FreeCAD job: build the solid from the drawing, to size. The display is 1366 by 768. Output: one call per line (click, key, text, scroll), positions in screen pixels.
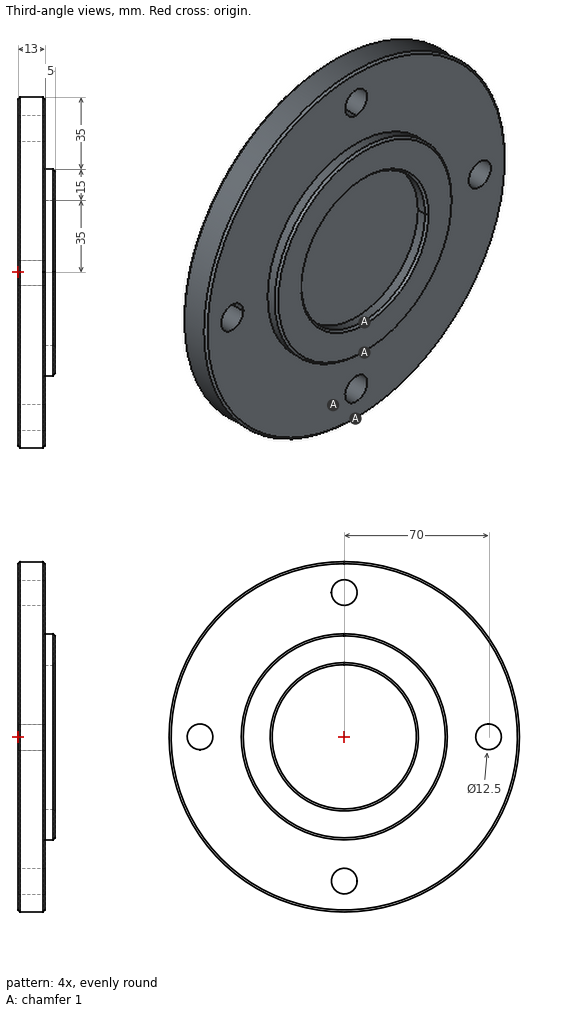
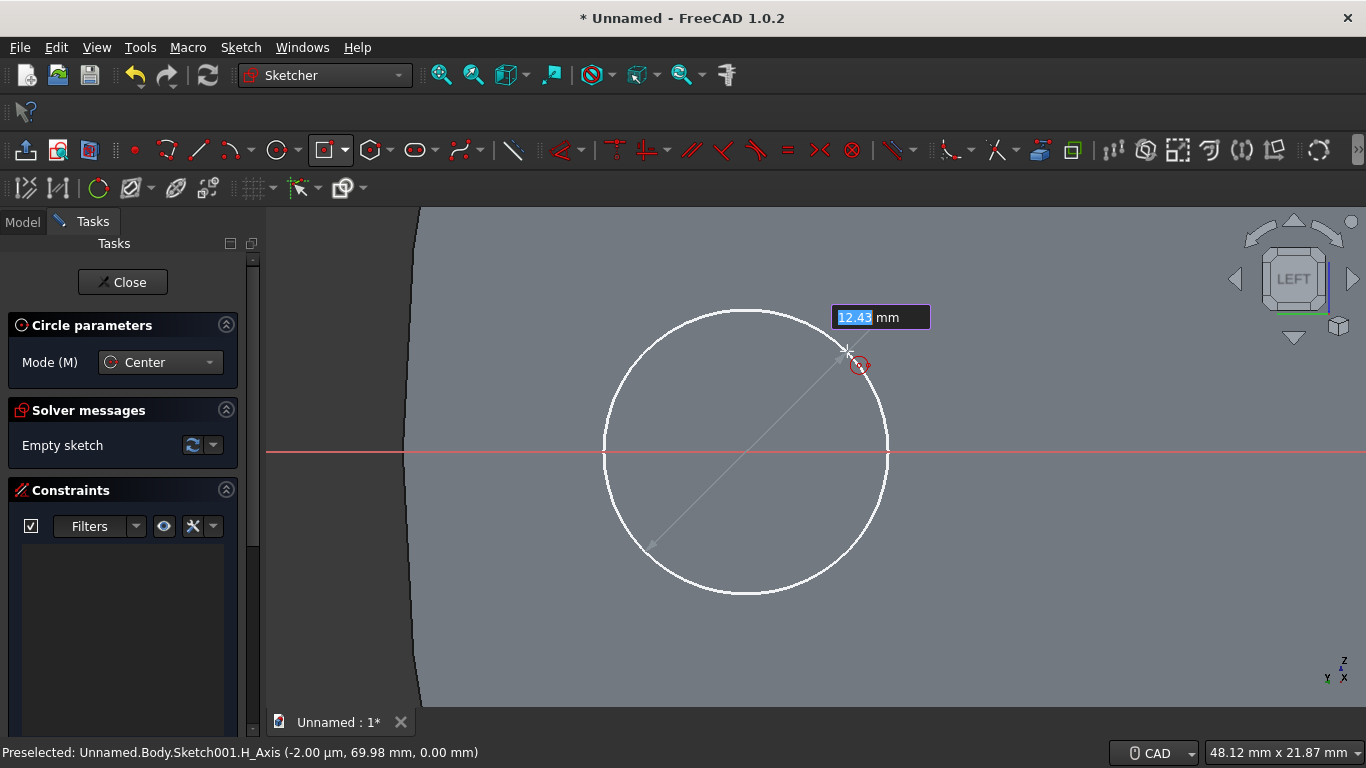
text(12.5)
key(Return)
key(Escape)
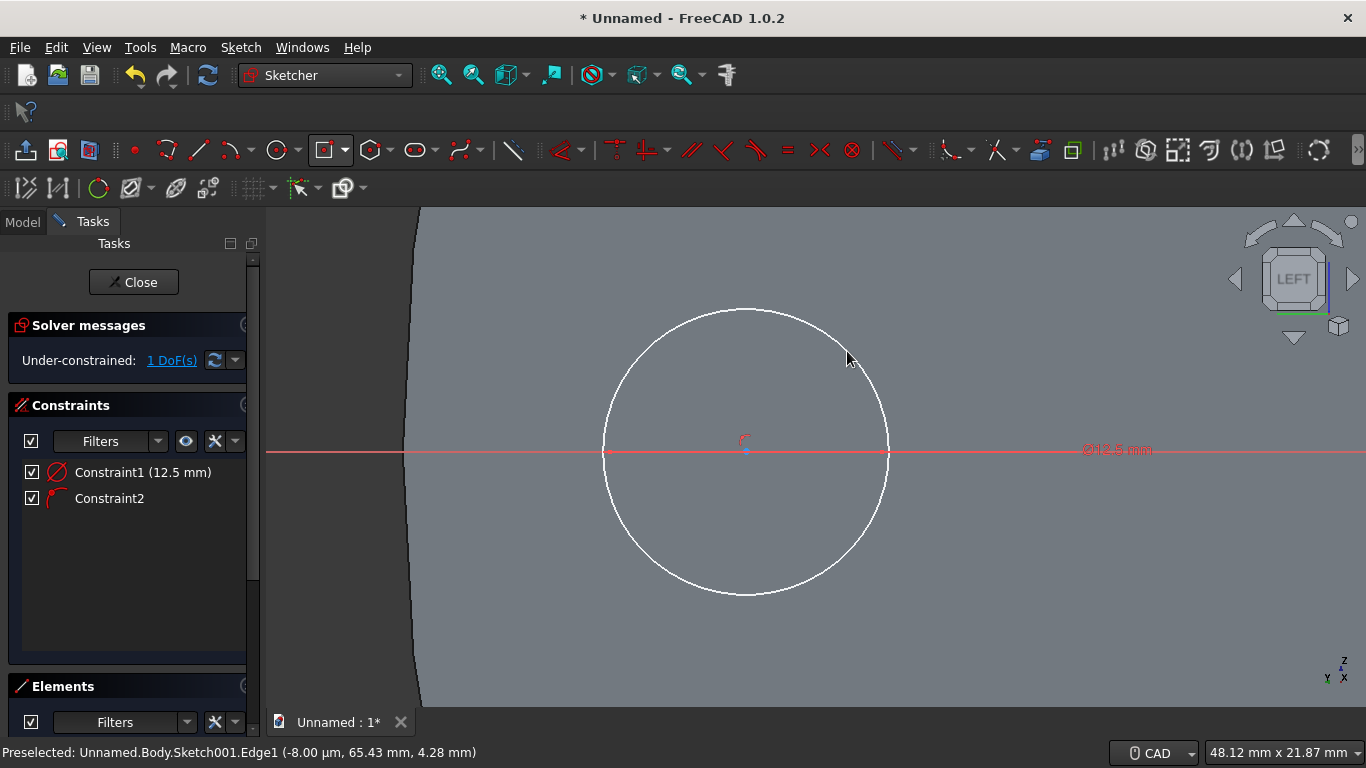
click(560, 150)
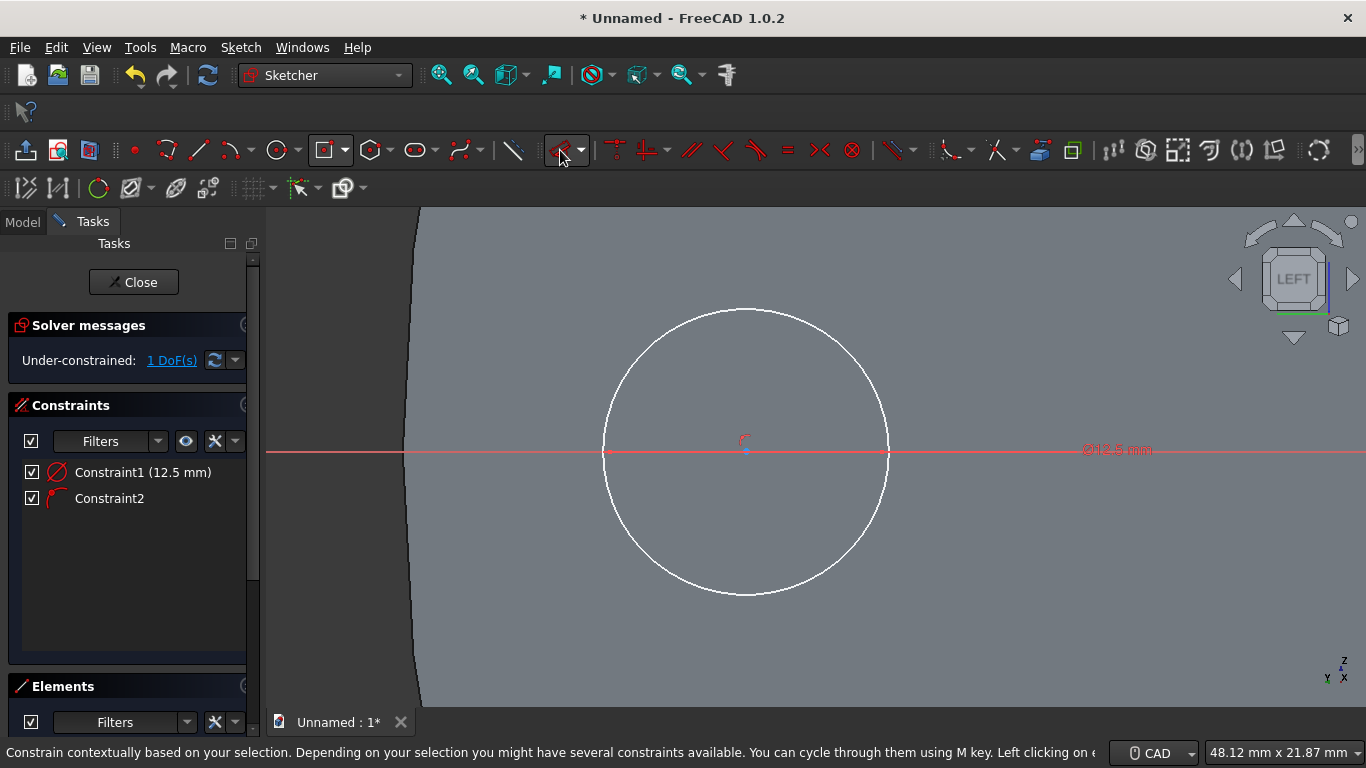
click(746, 452)
click(973, 486)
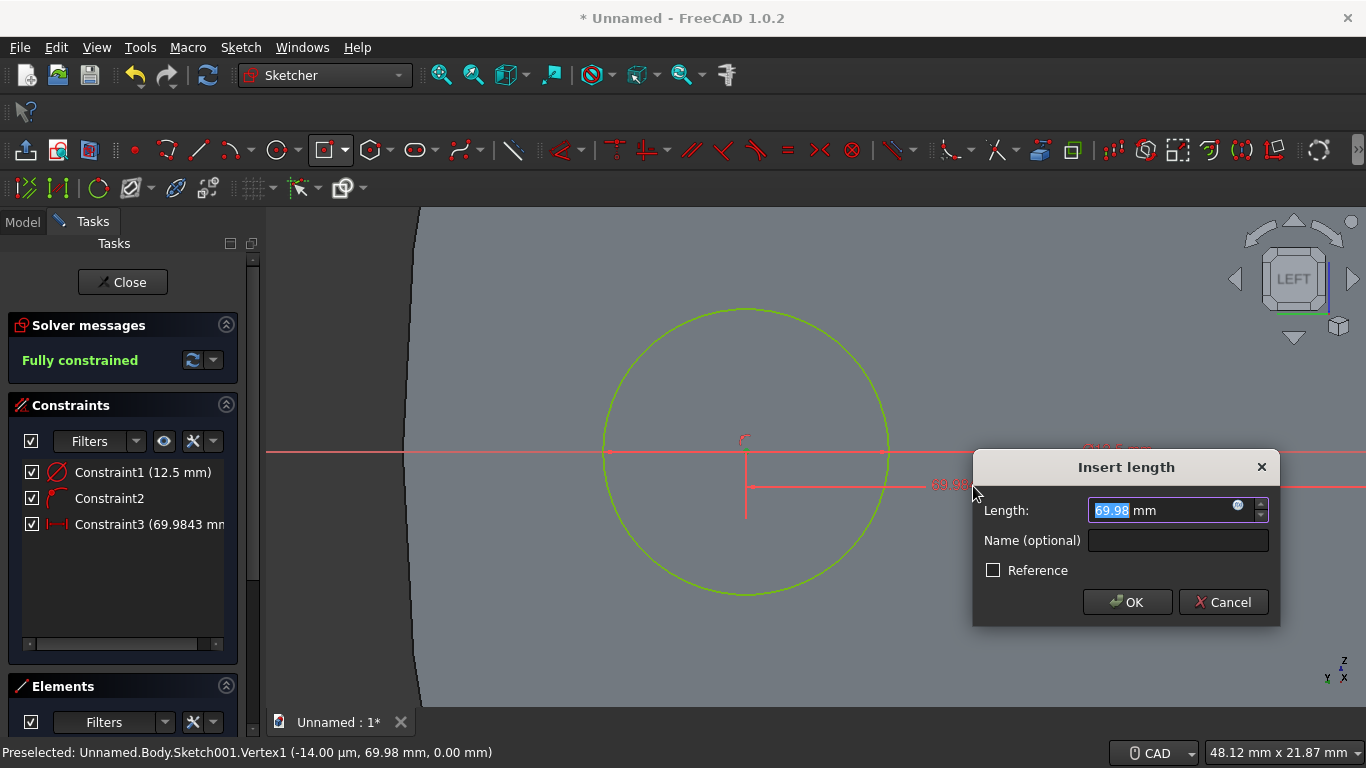
text(70)
key(Return)
key(Escape)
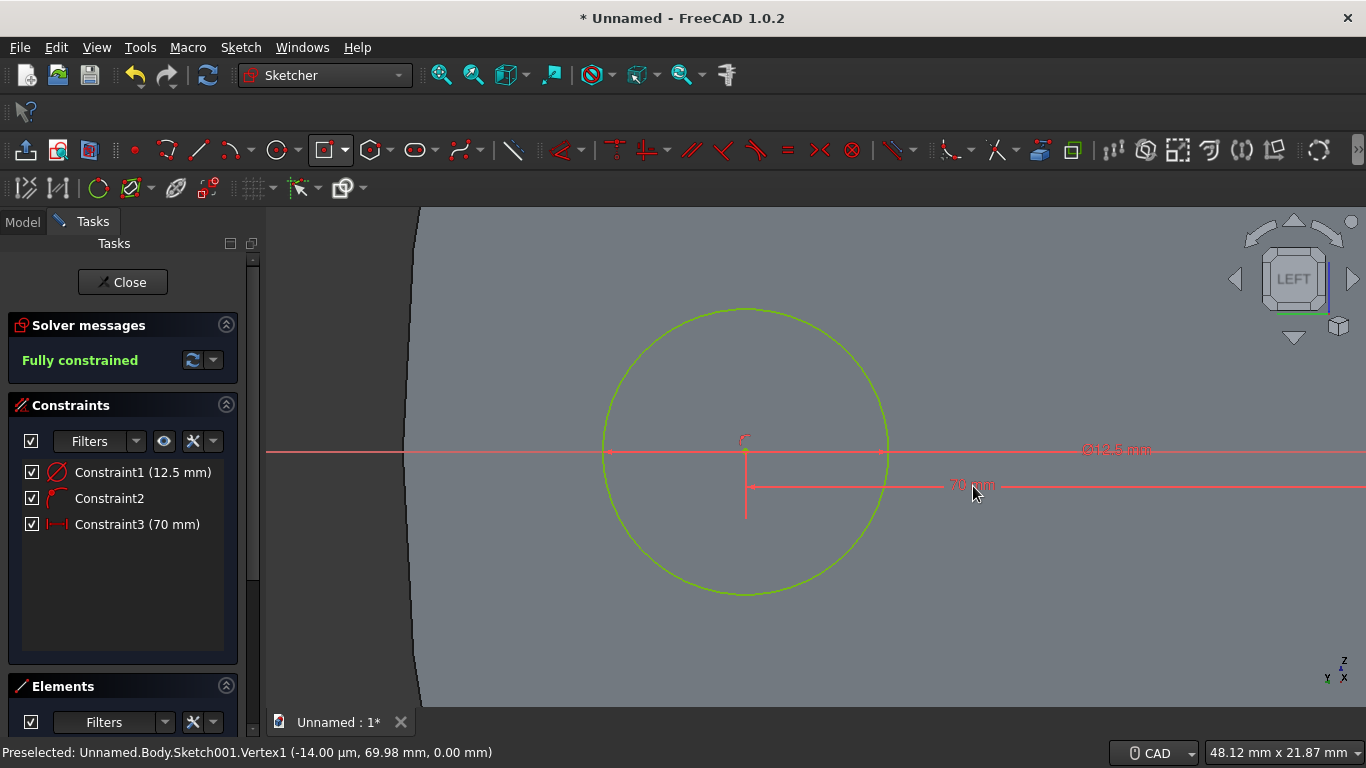
click(123, 282)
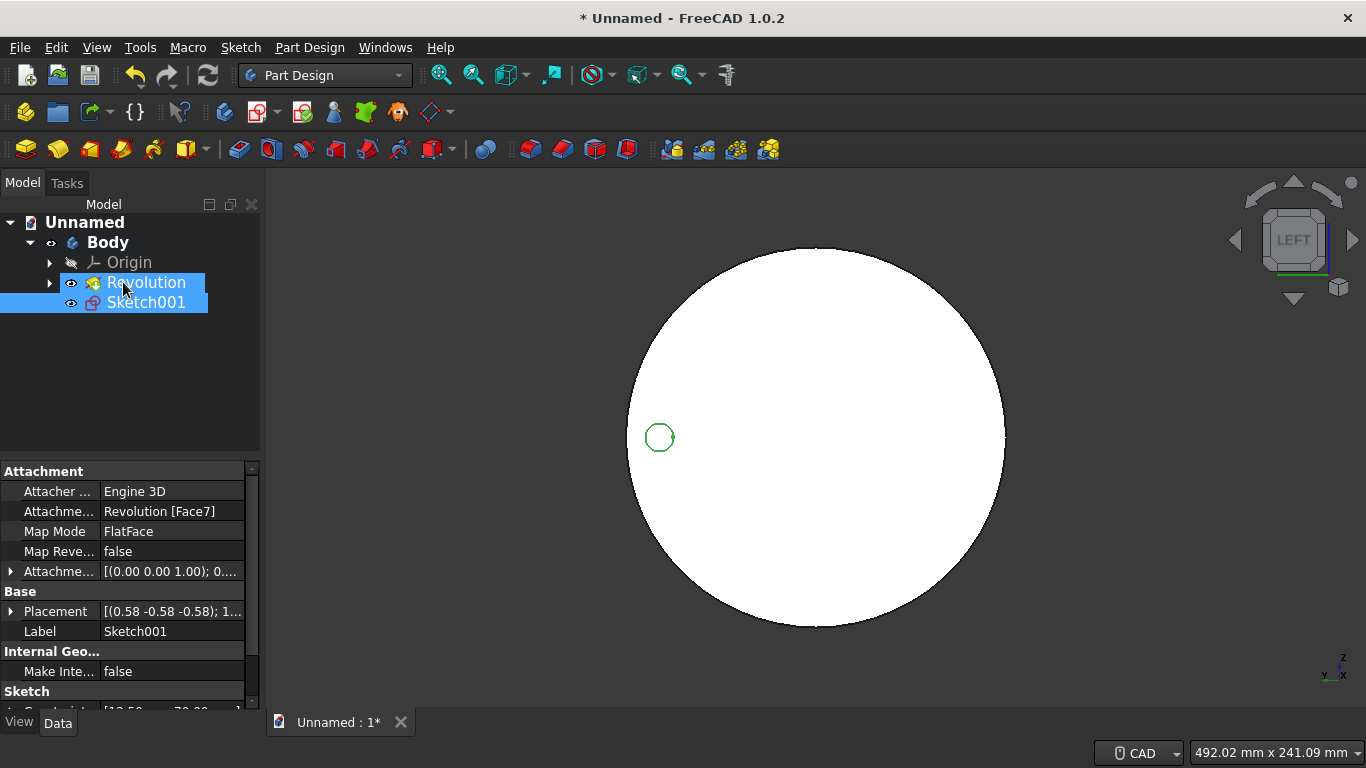
click(240, 150)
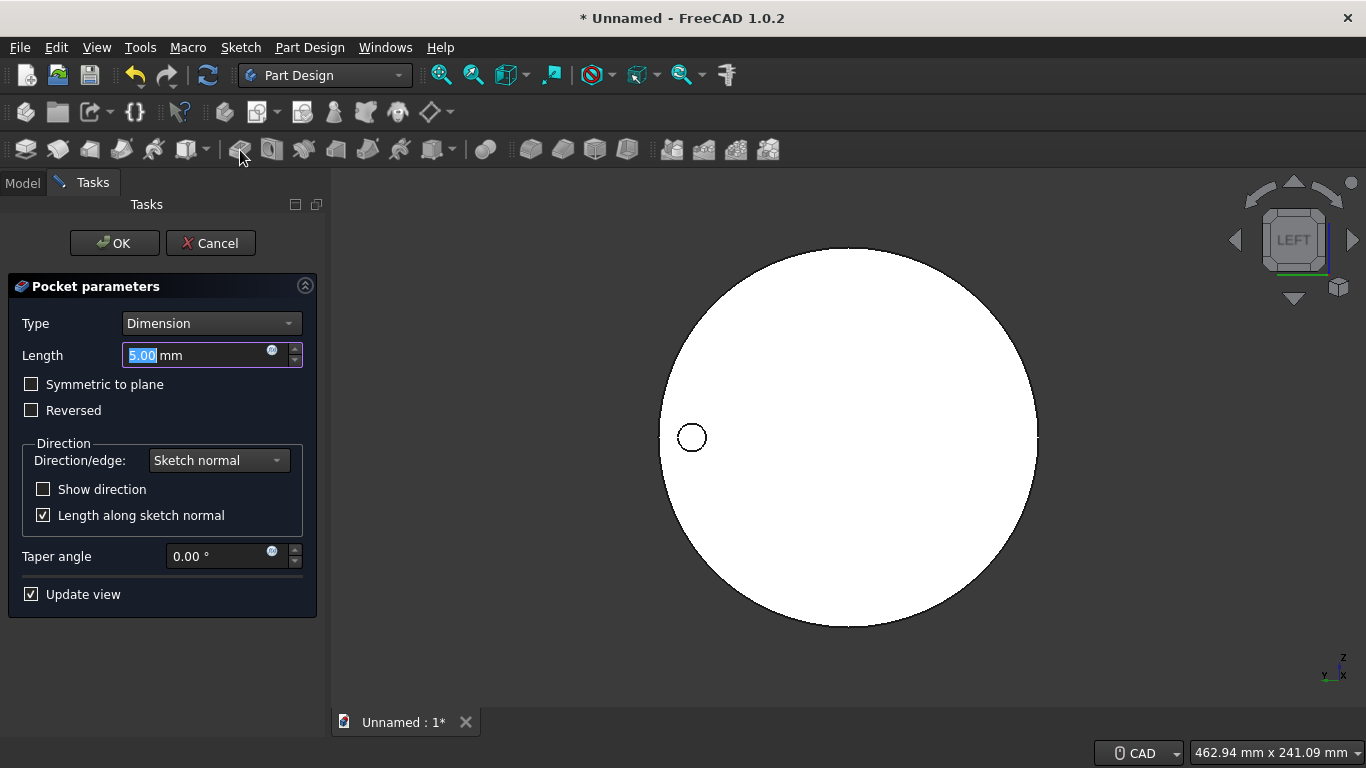
click(212, 324)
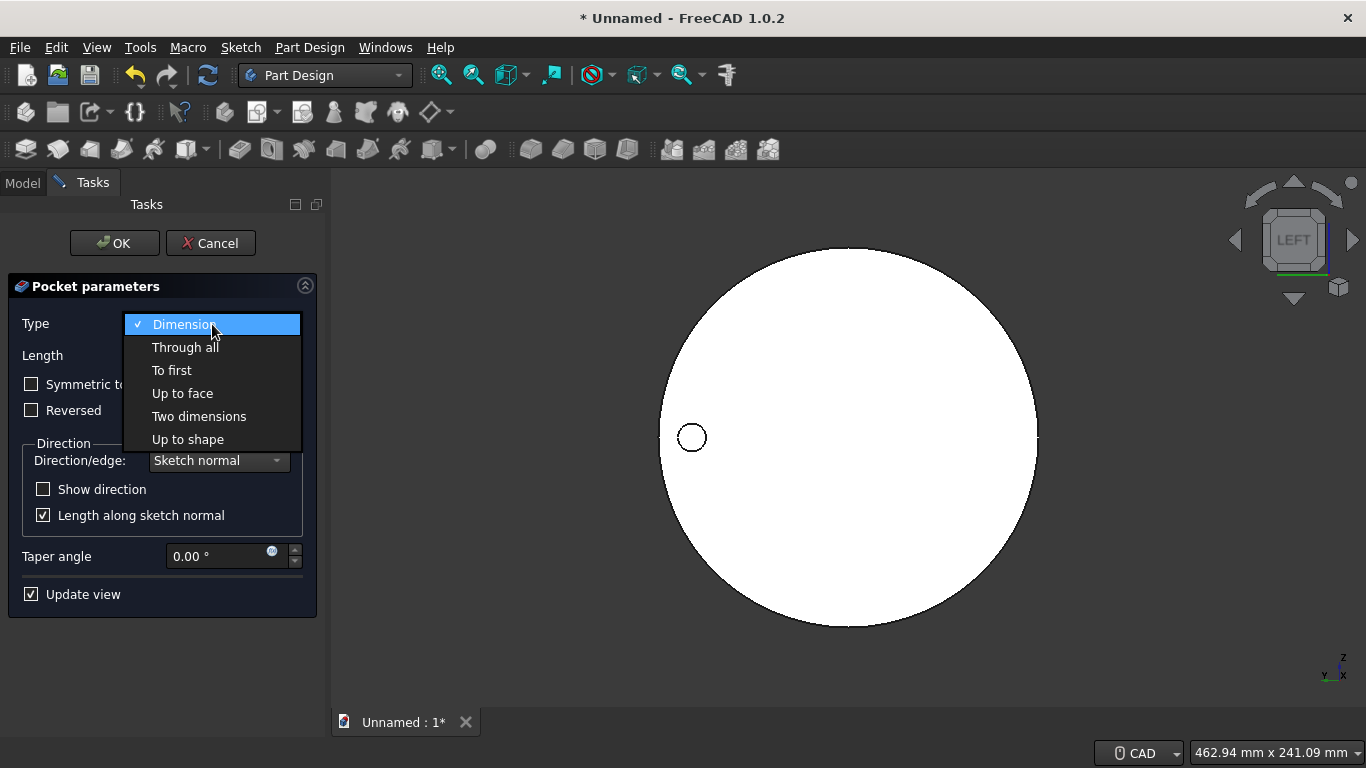
click(212, 348)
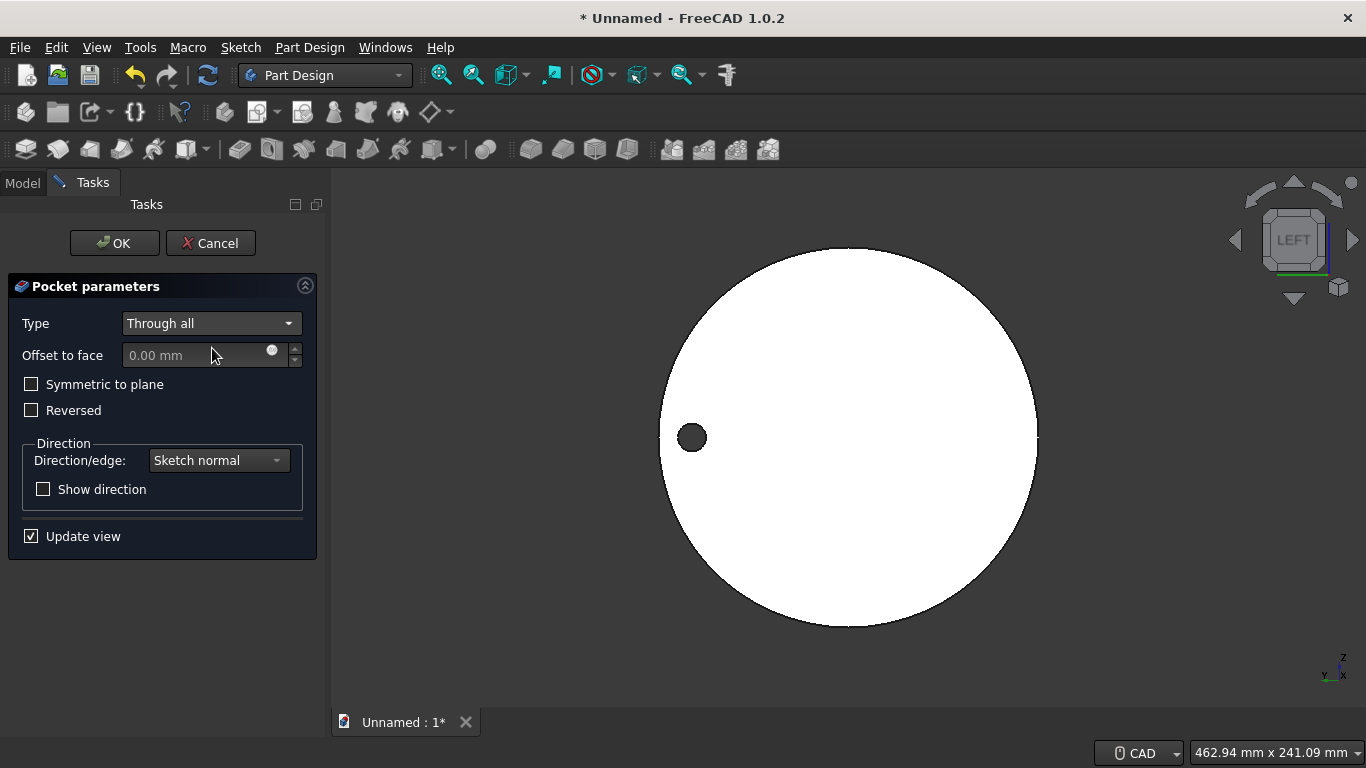
click(115, 243)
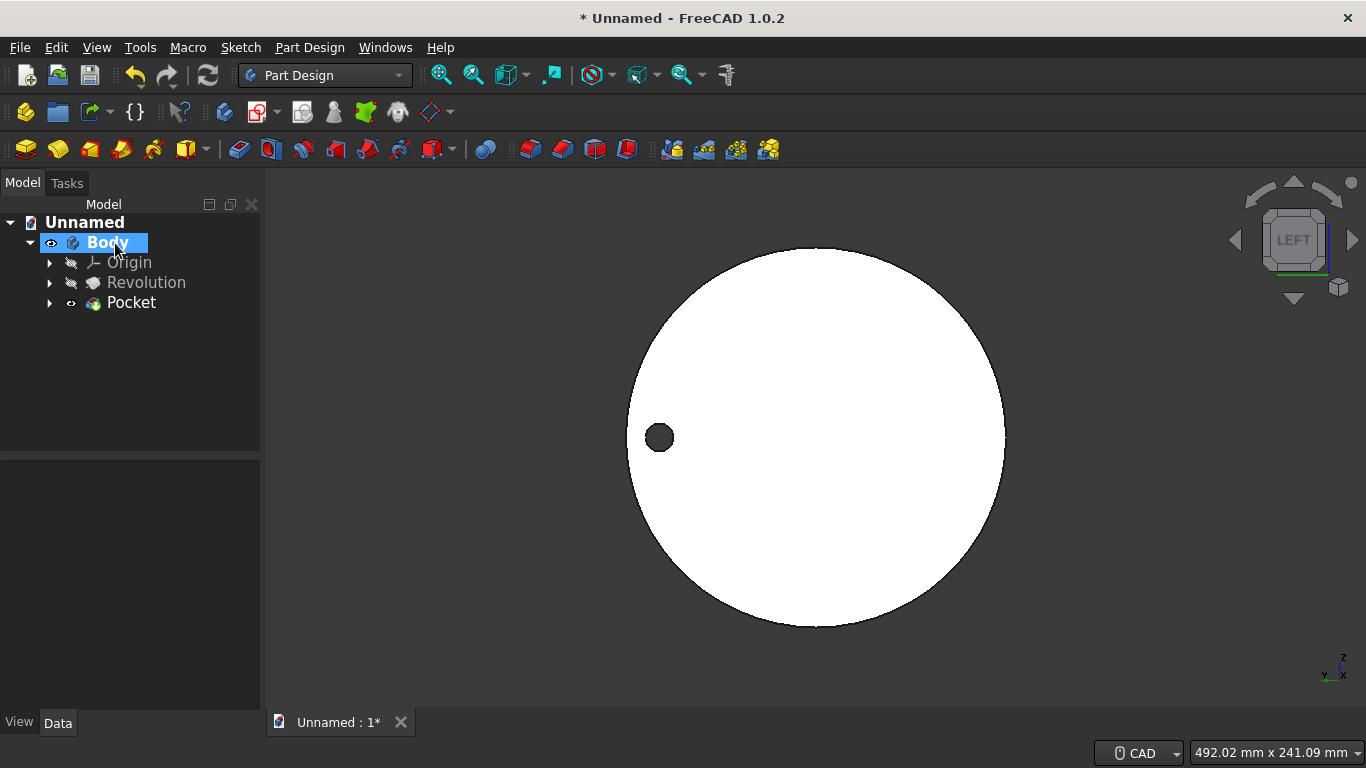
click(116, 303)